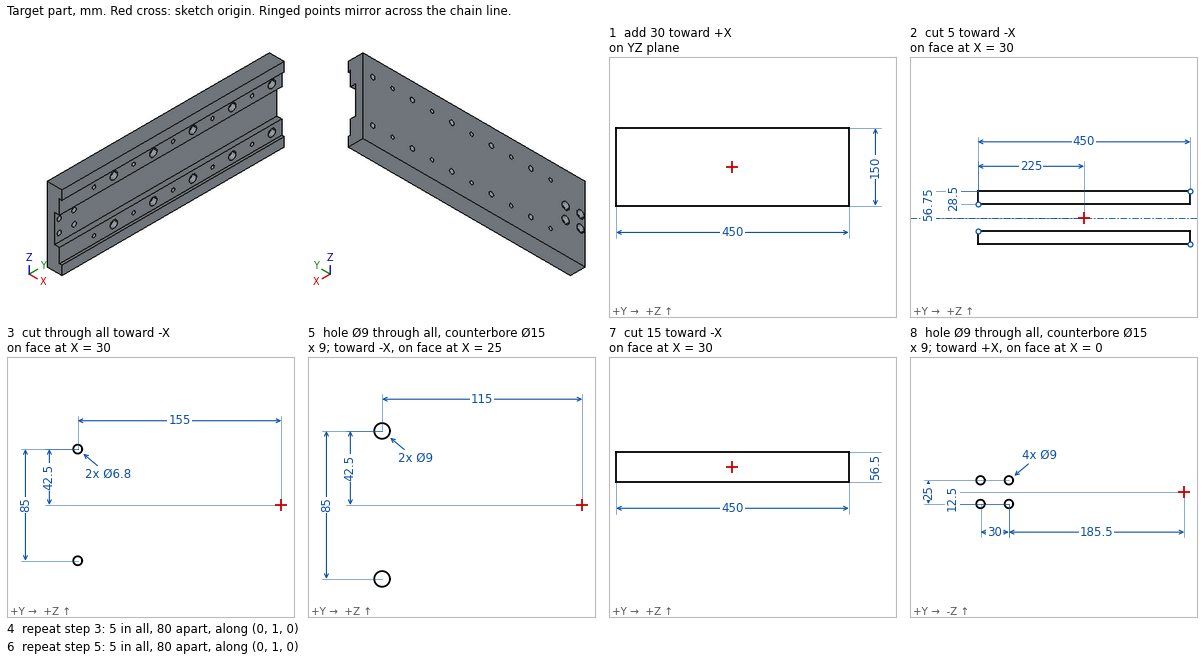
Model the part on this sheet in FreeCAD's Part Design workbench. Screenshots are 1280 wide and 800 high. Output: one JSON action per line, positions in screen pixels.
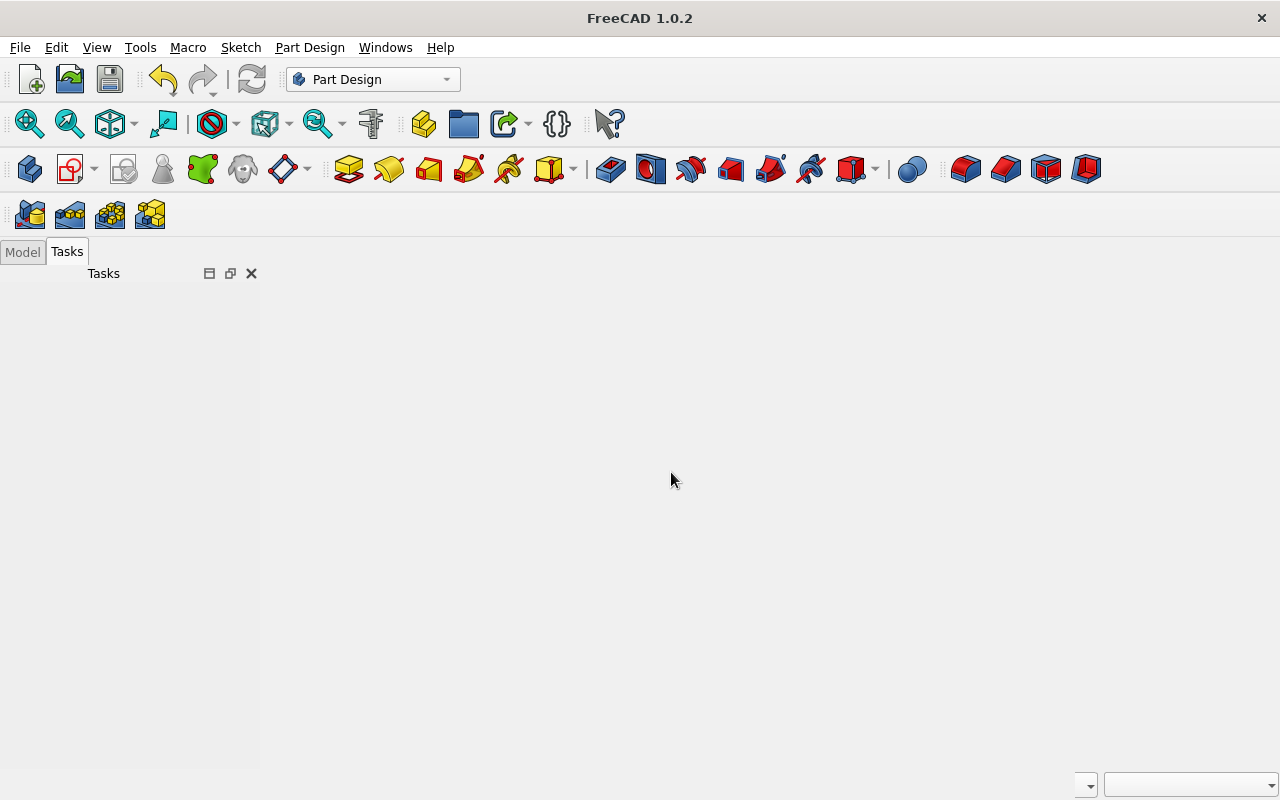
{"action": "left_click", "coordinate": [30, 80]}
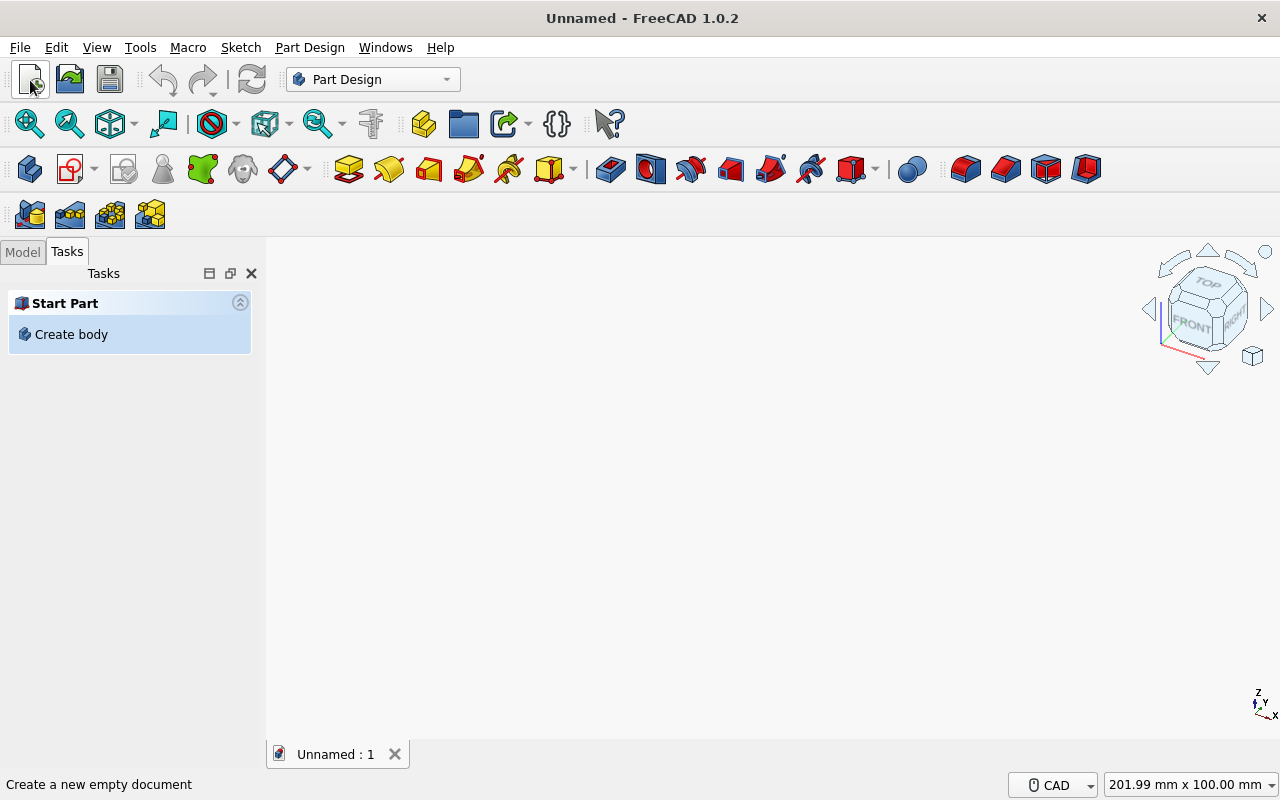
{"action": "left_click", "coordinate": [70, 170]}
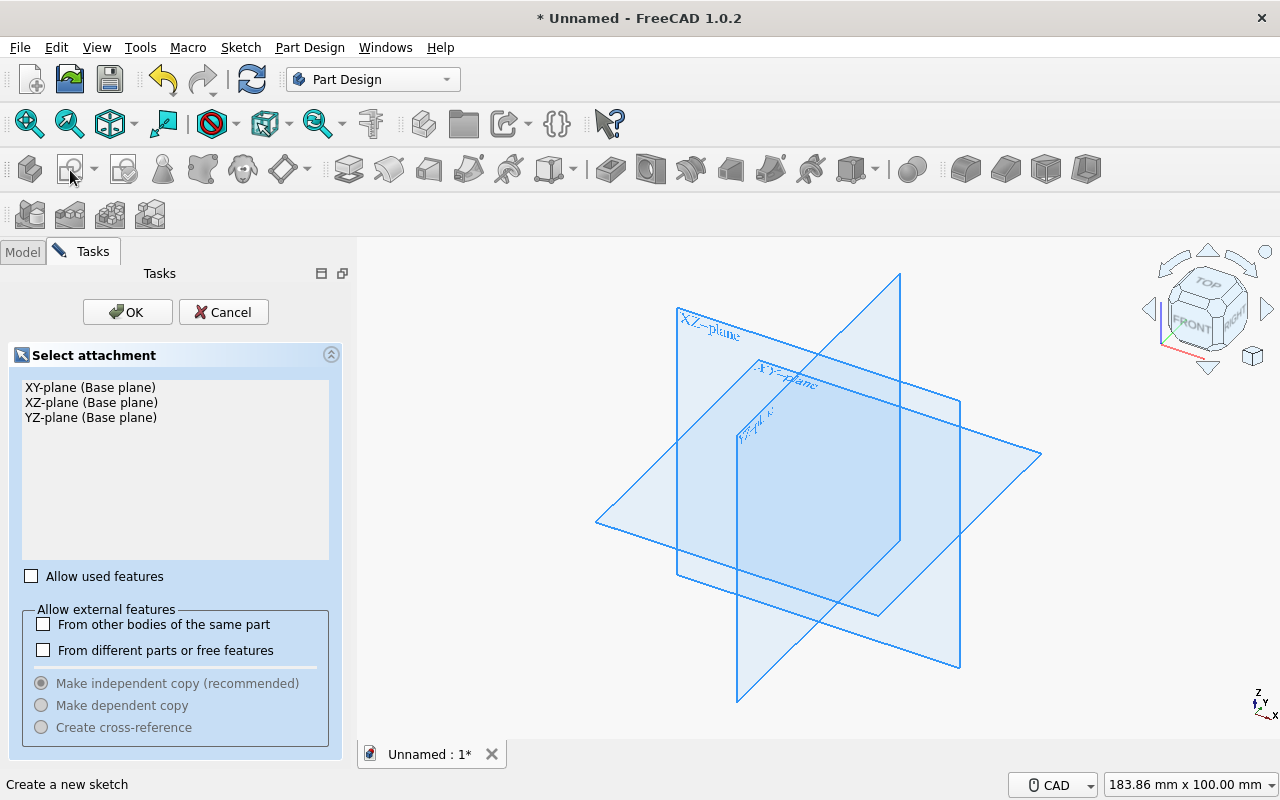
{"action": "left_click", "coordinate": [82, 418]}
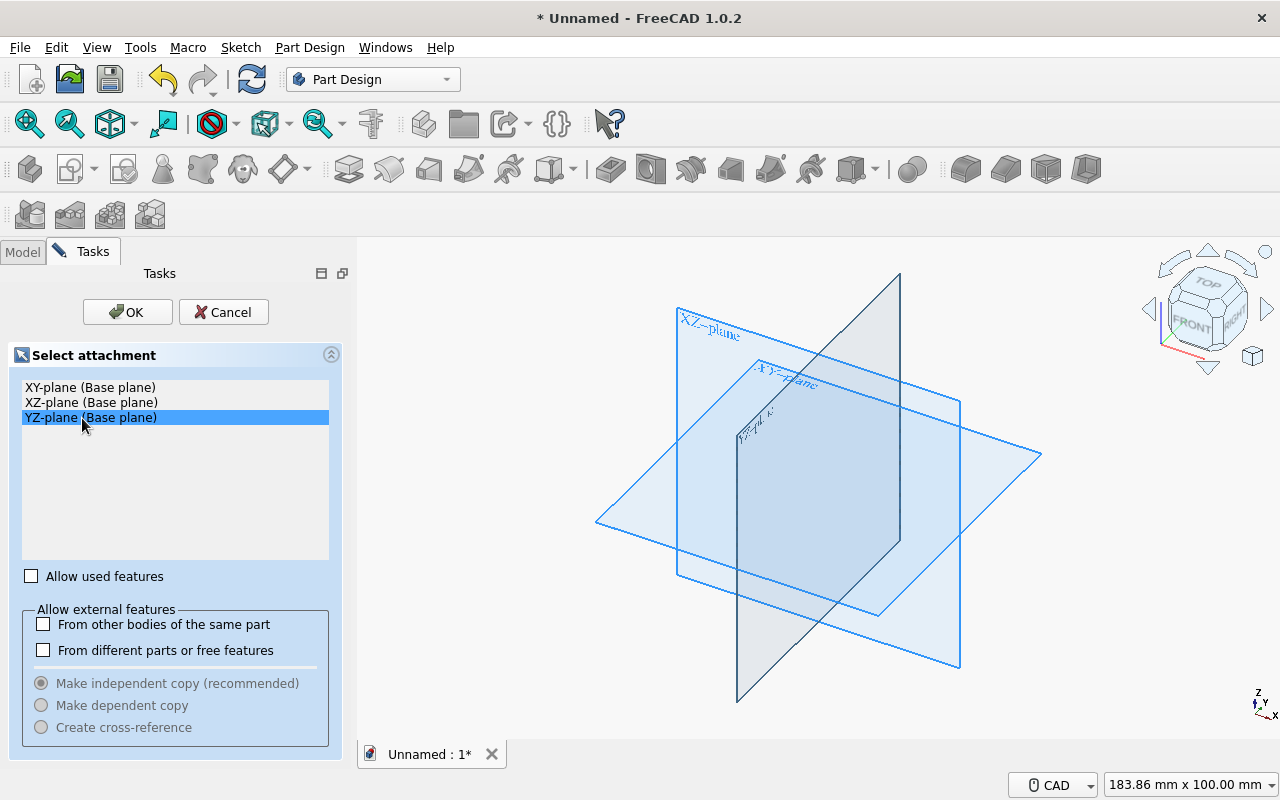
{"action": "left_click", "coordinate": [128, 312]}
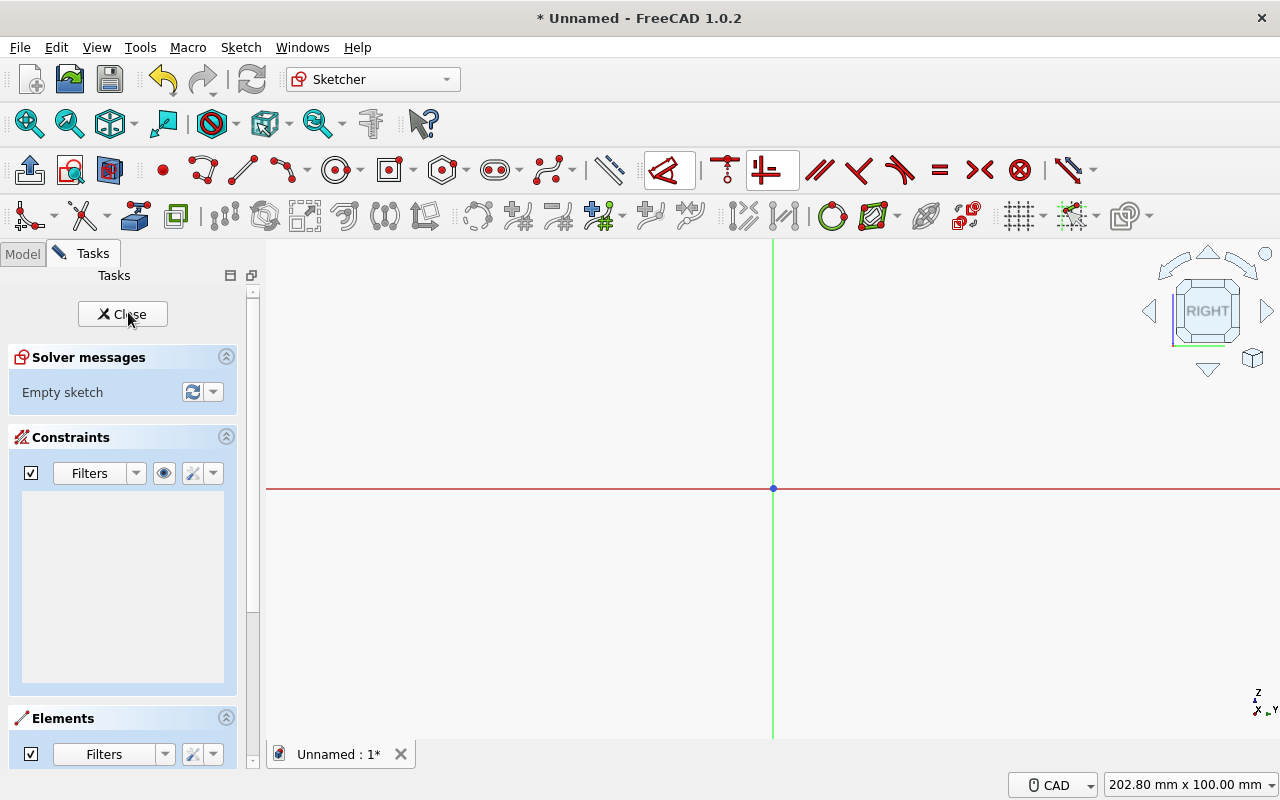
{"action": "scroll", "coordinate": [682, 489], "scroll_direction": "down", "scroll_amount": 7}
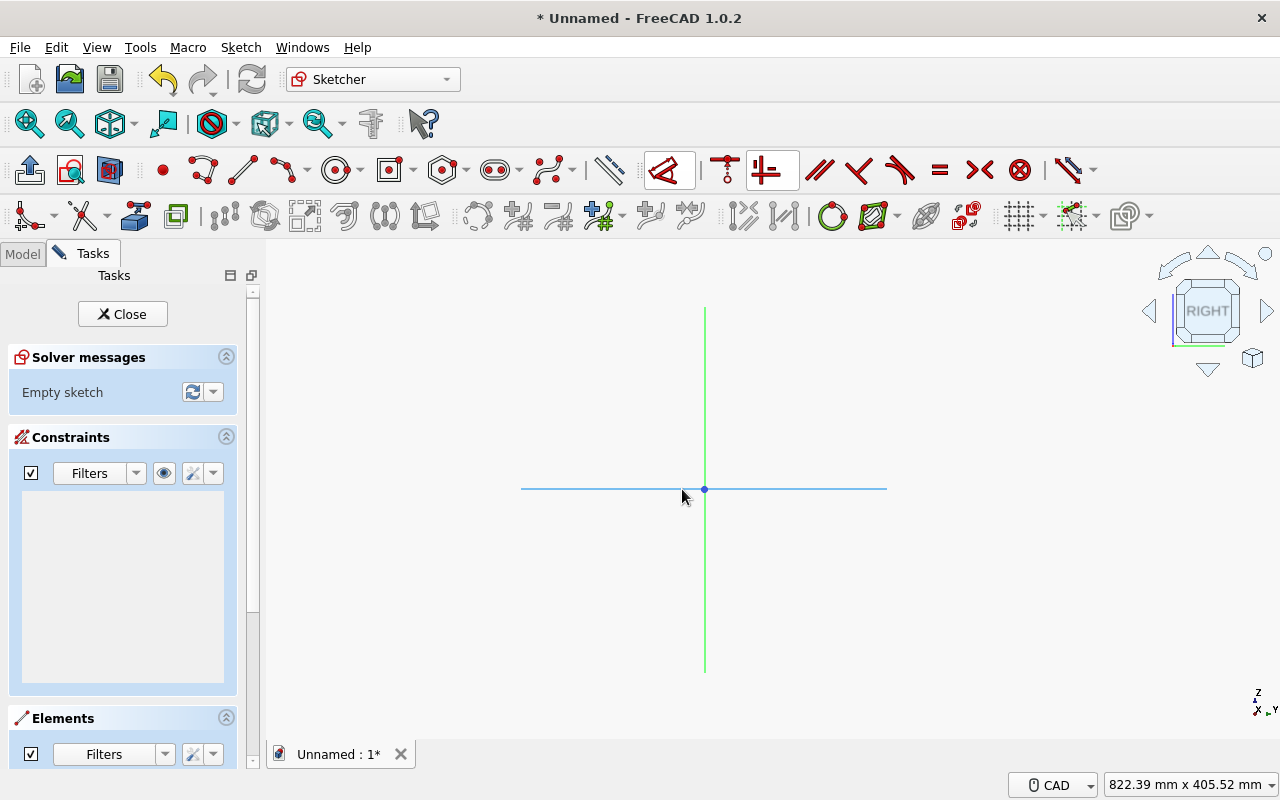
{"action": "left_click", "coordinate": [390, 170]}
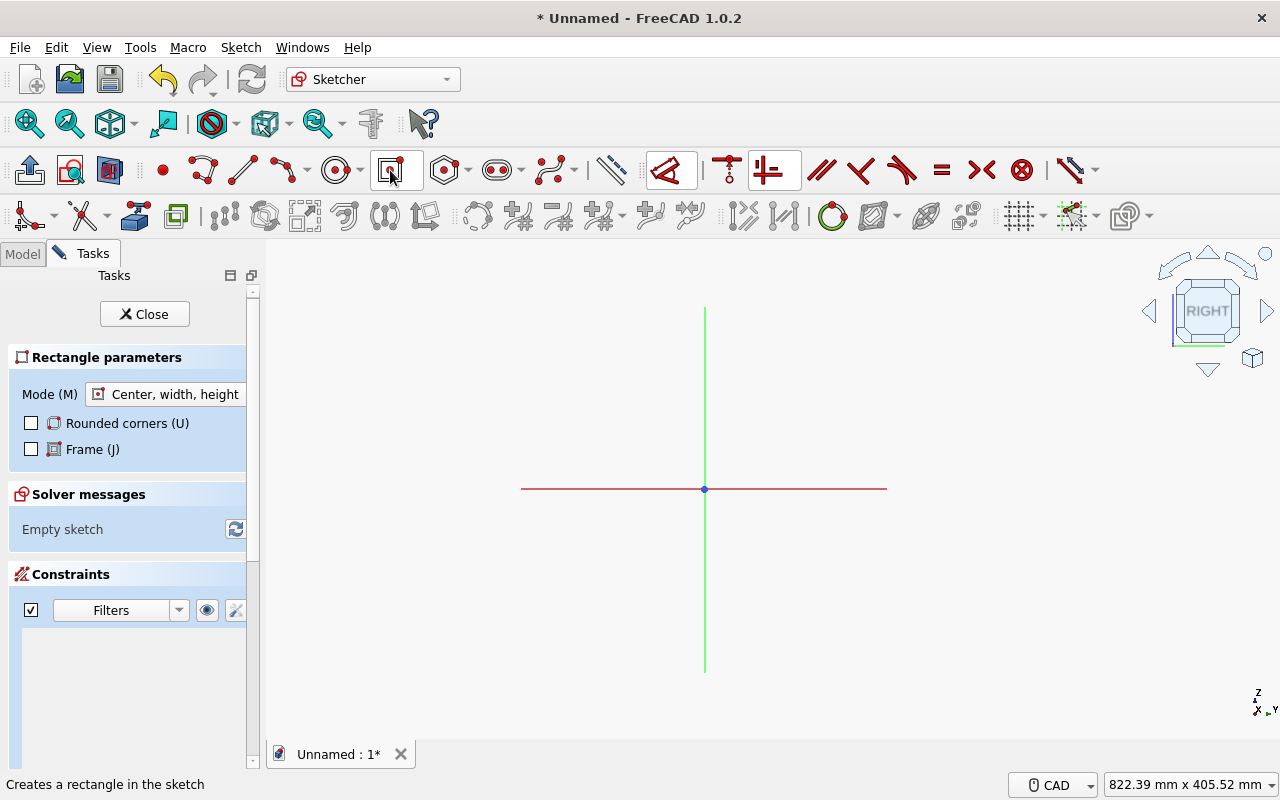
{"action": "left_click", "coordinate": [705, 489]}
{"action": "left_click", "coordinate": [982, 397]}
{"action": "key", "text": "Escape"}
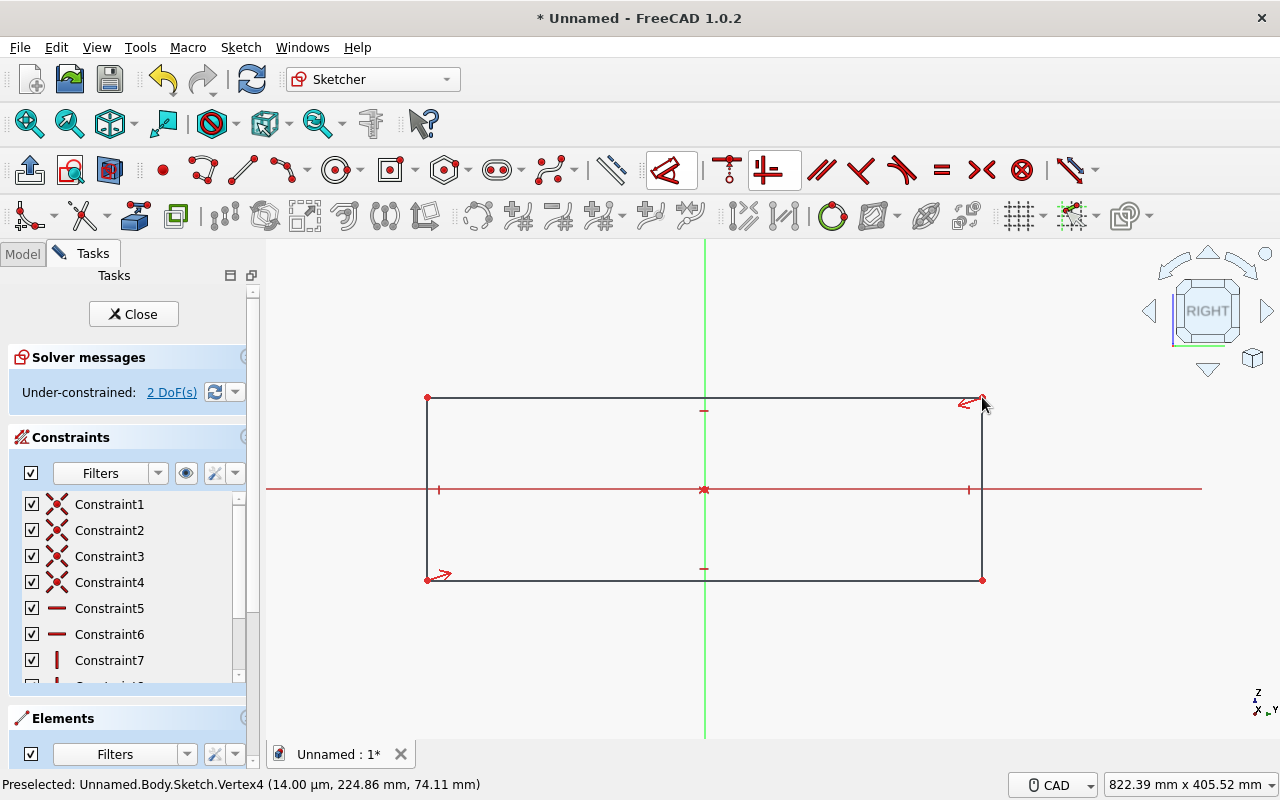
{"action": "left_click", "coordinate": [666, 170]}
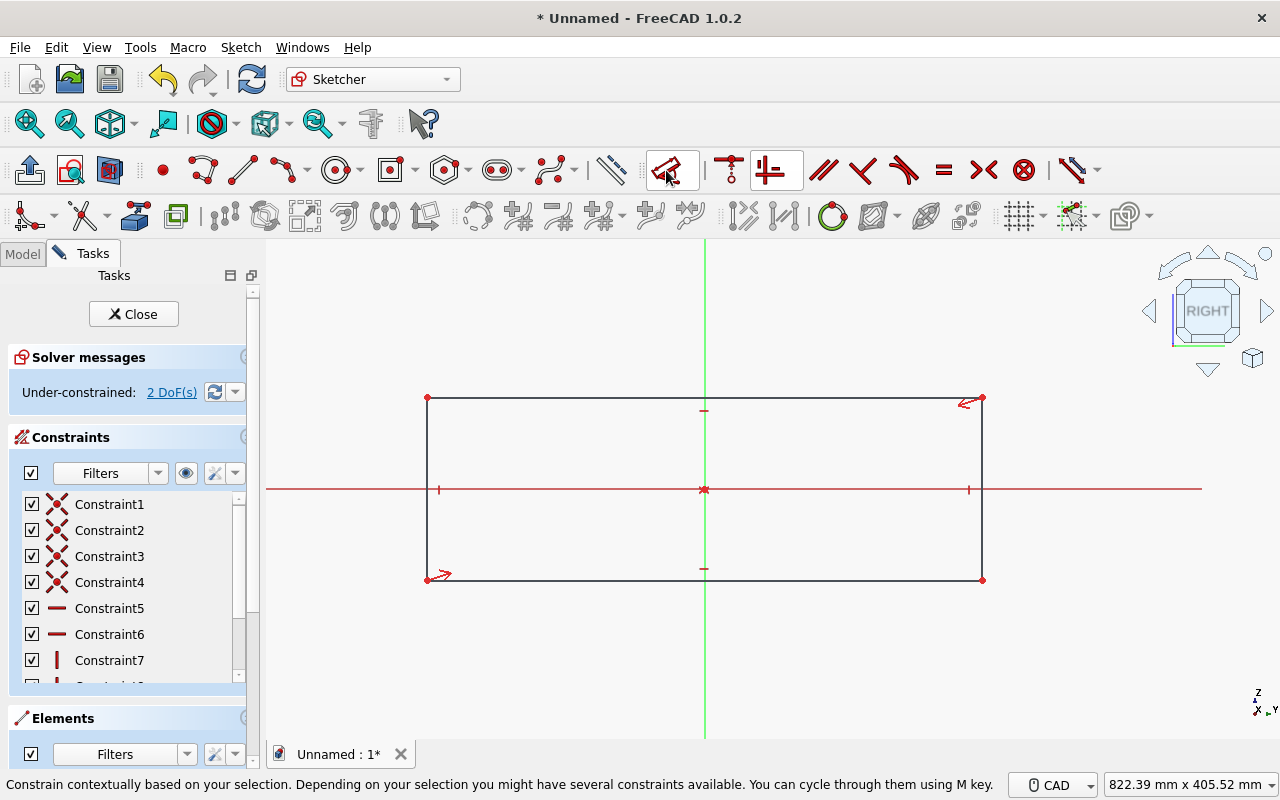
{"action": "left_click", "coordinate": [594, 581]}
{"action": "left_click", "coordinate": [577, 615]}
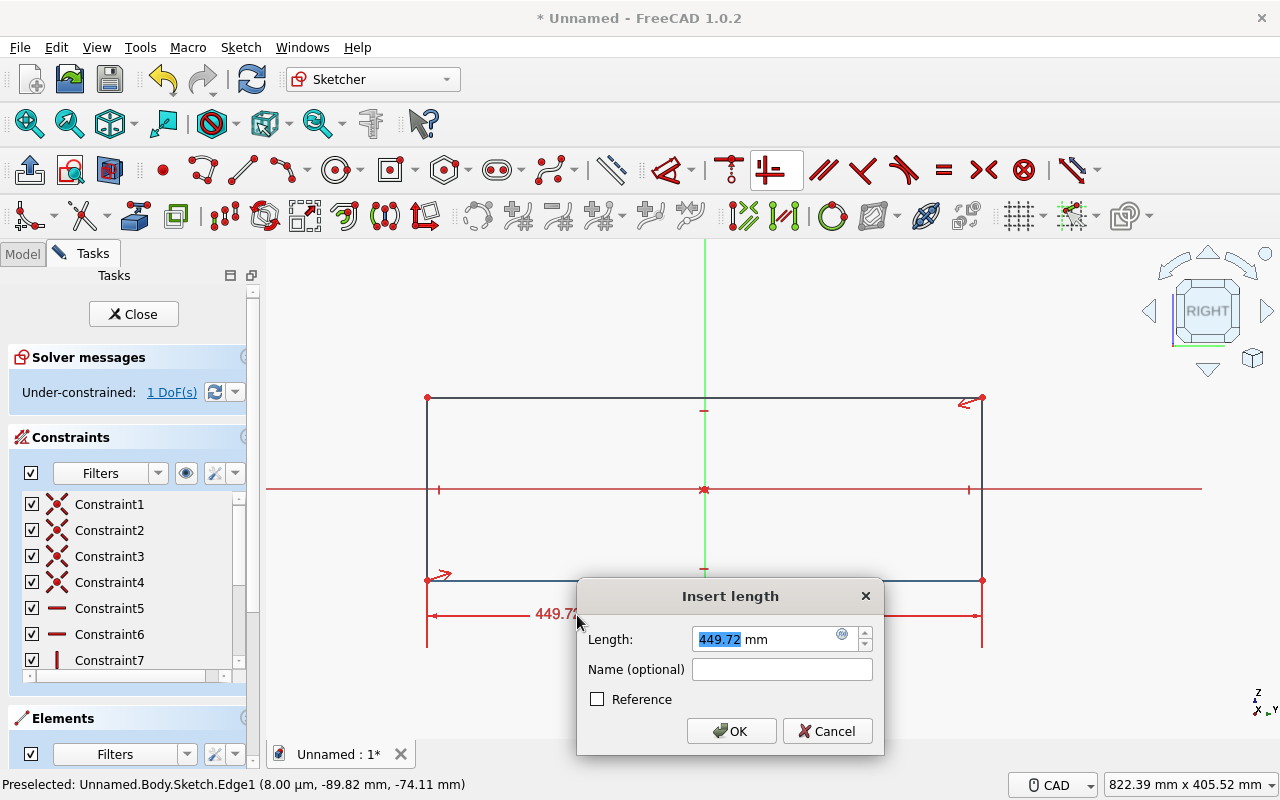
{"action": "type", "text": "450"}
{"action": "key", "text": "Return"}